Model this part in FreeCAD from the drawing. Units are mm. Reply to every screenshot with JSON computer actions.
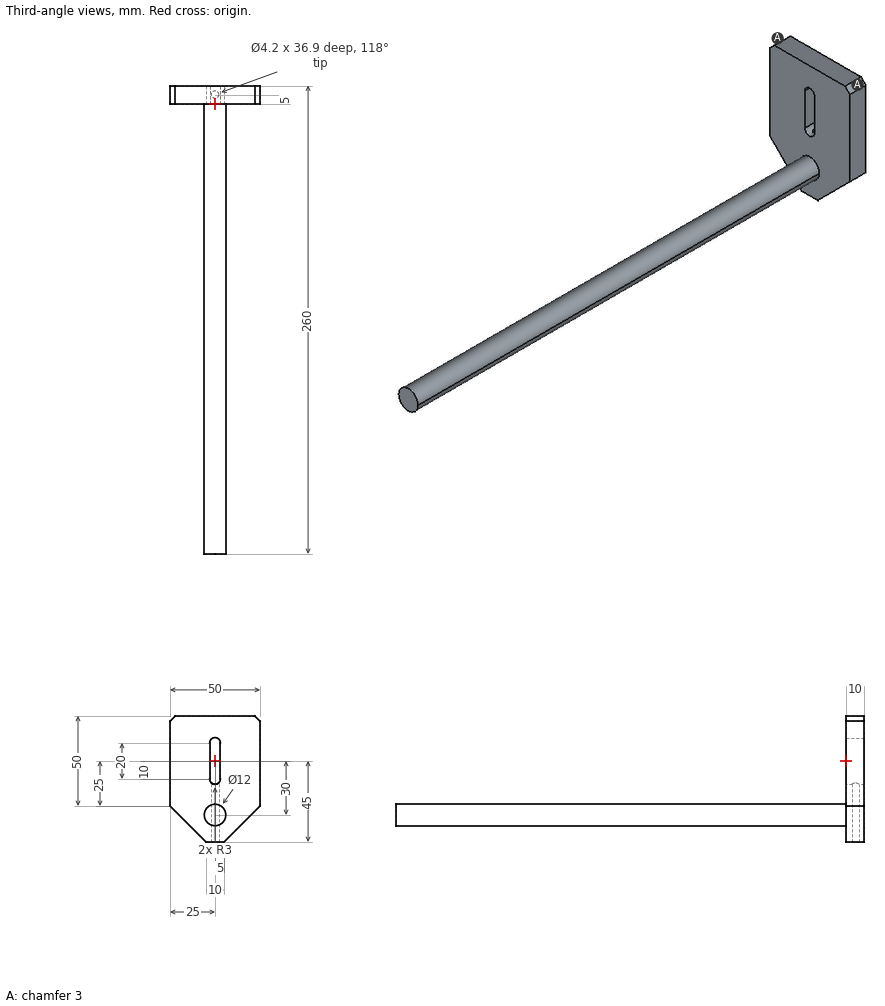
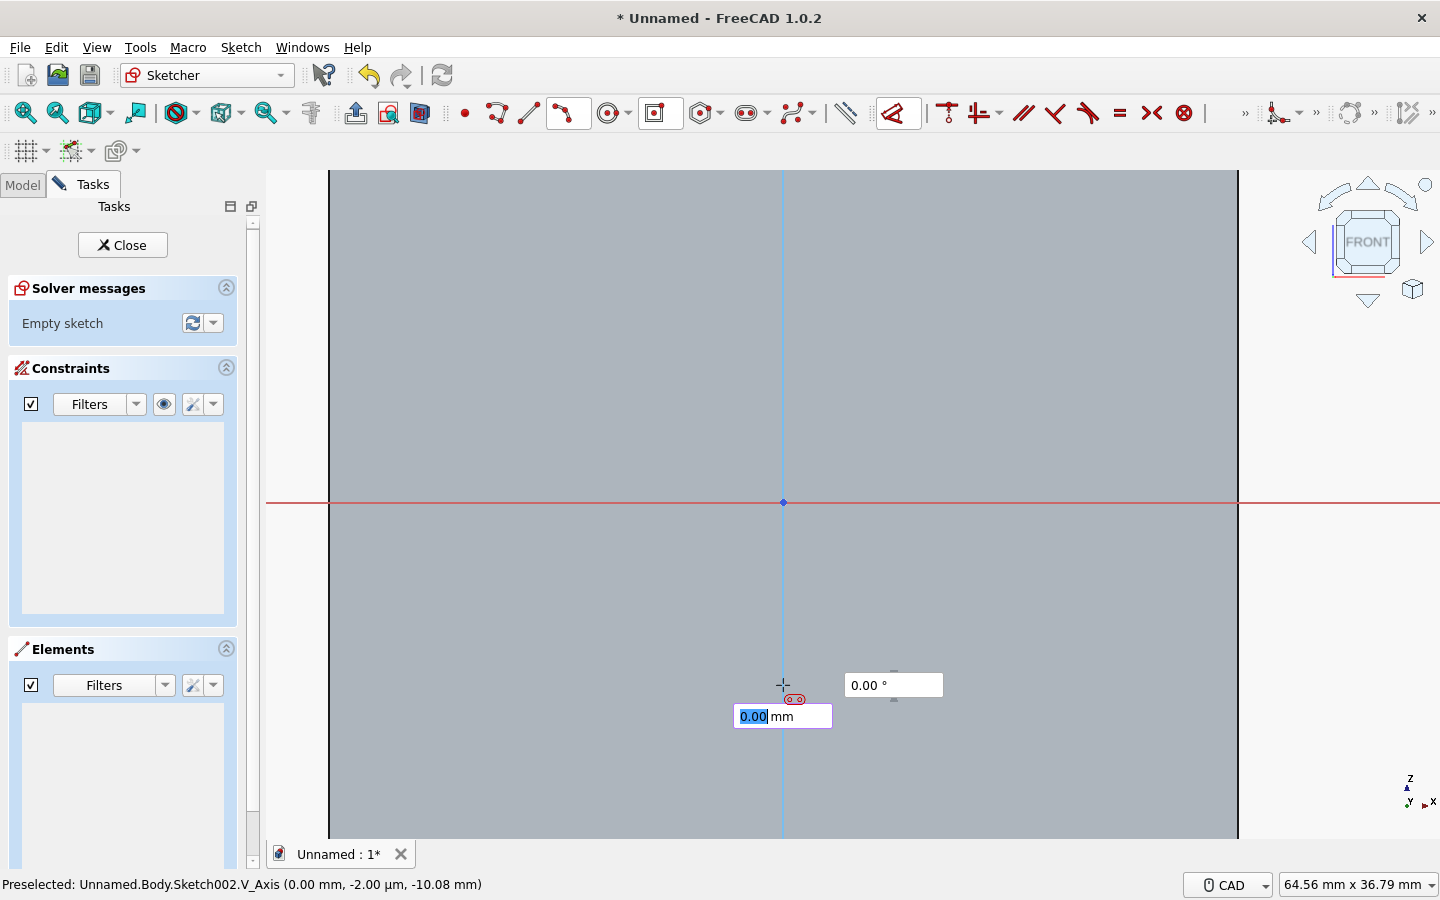
{"action": "left_click", "coordinate": [792, 321]}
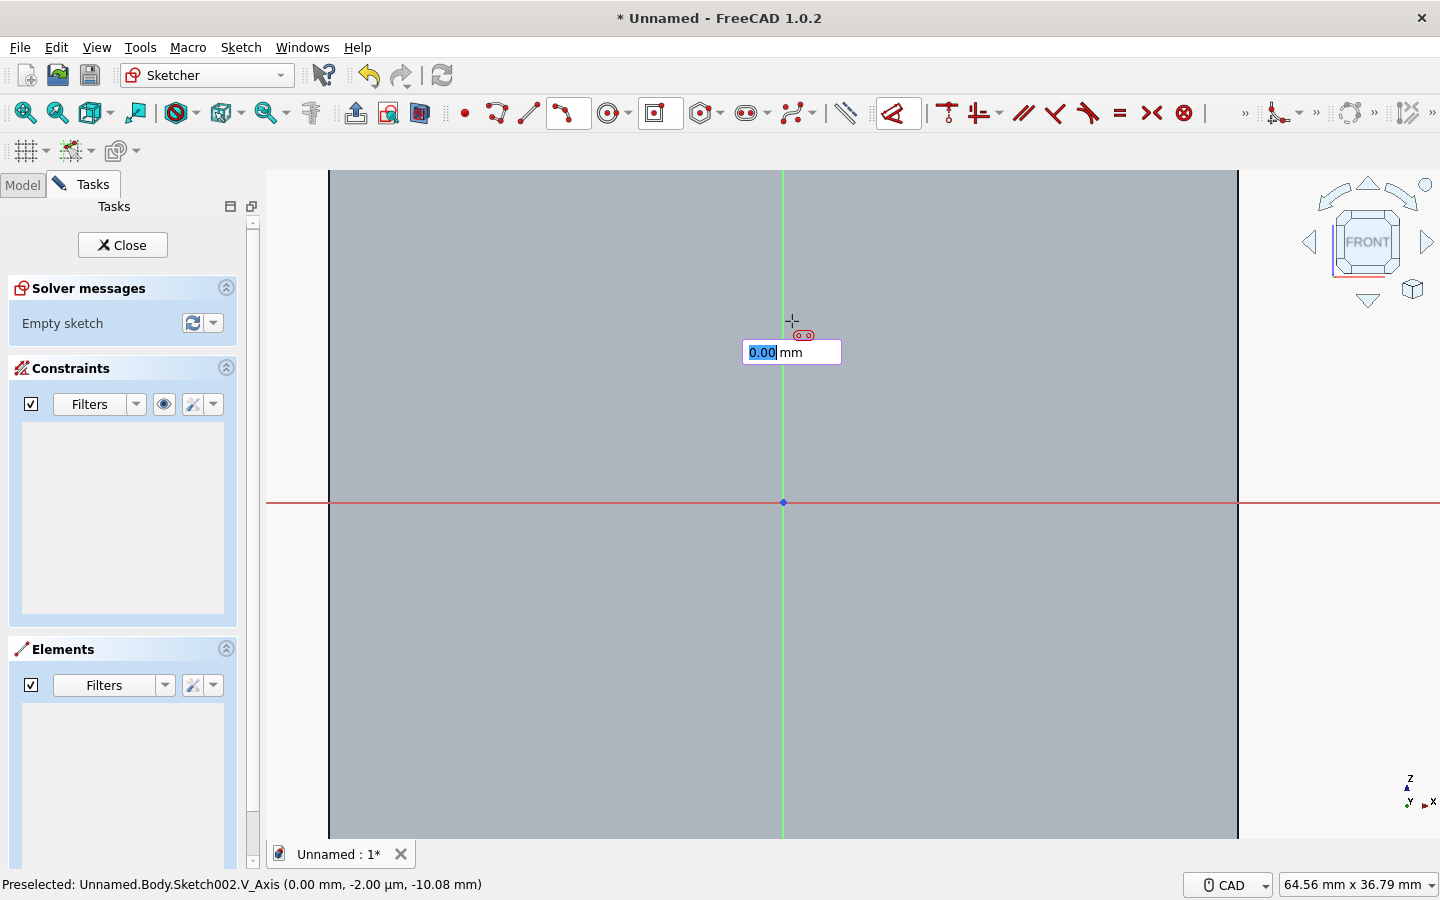
{"action": "left_click", "coordinate": [729, 448]}
{"action": "key", "text": "Escape"}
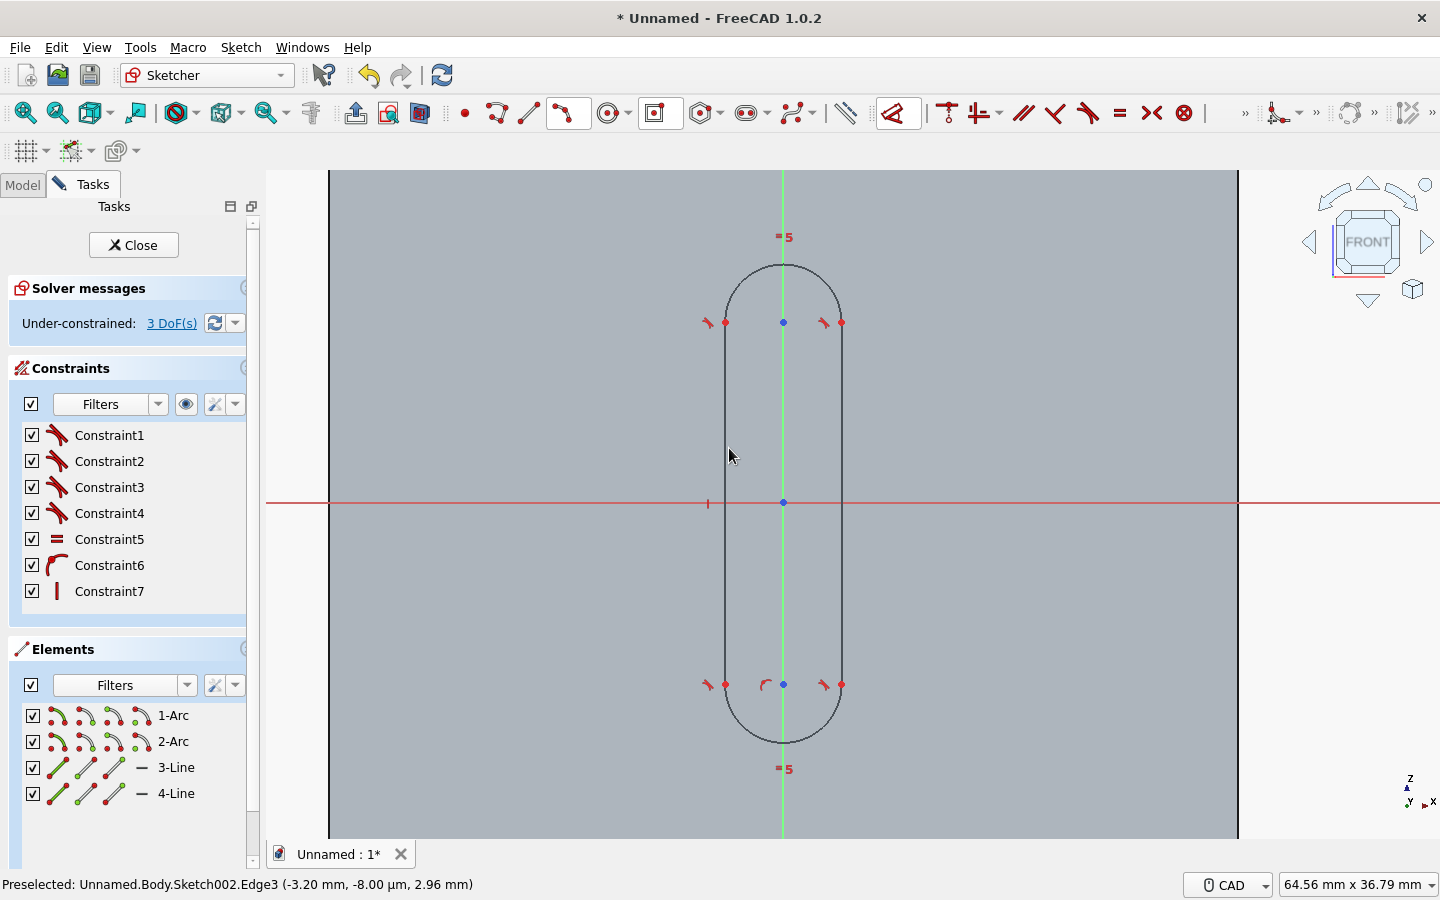
{"action": "left_click", "coordinate": [749, 732]}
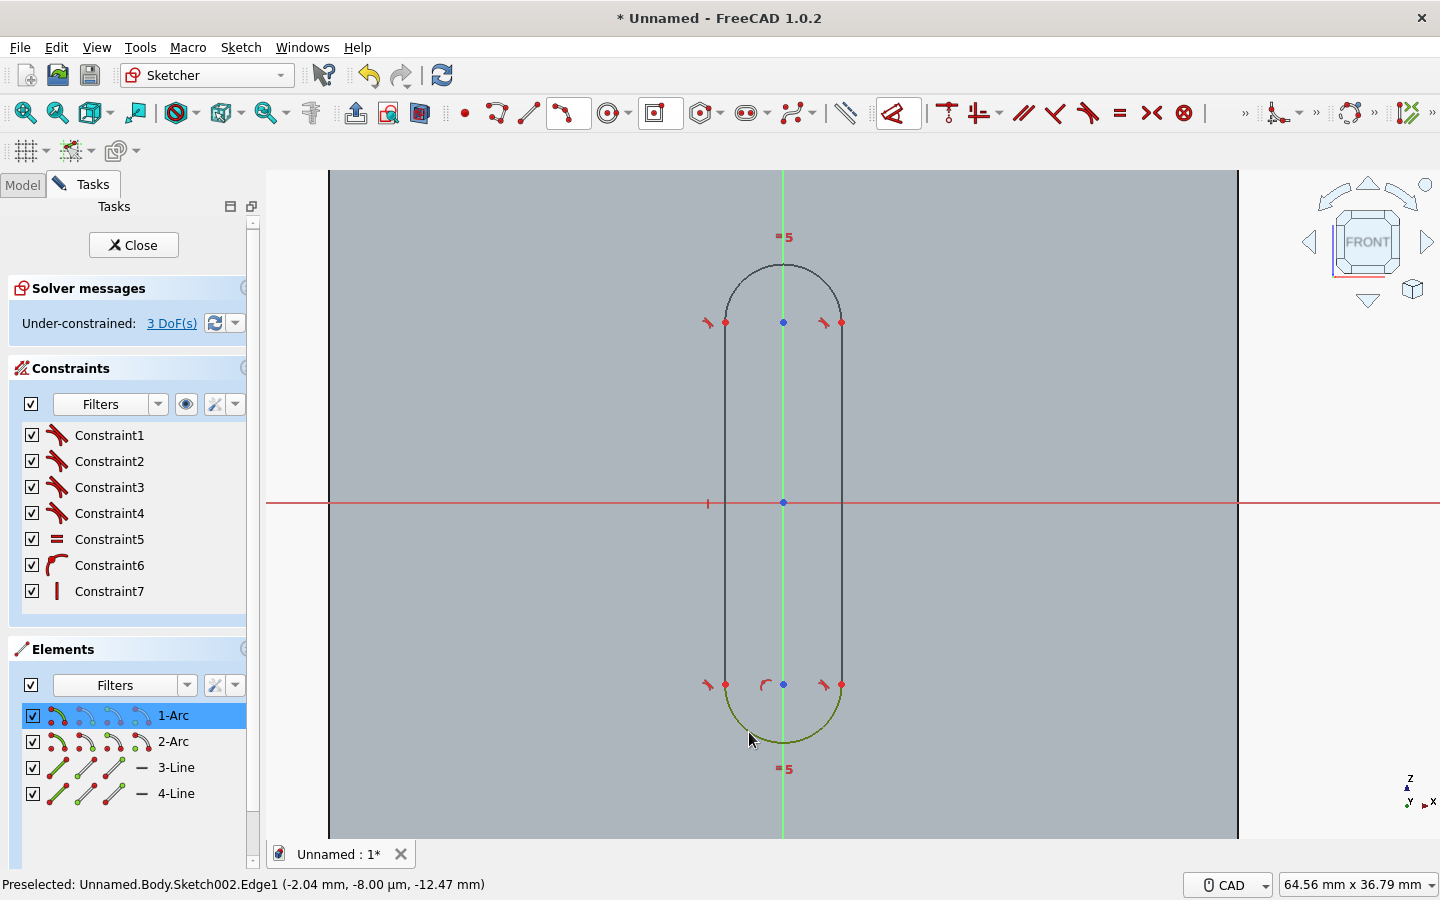
{"action": "key", "text": "k r"}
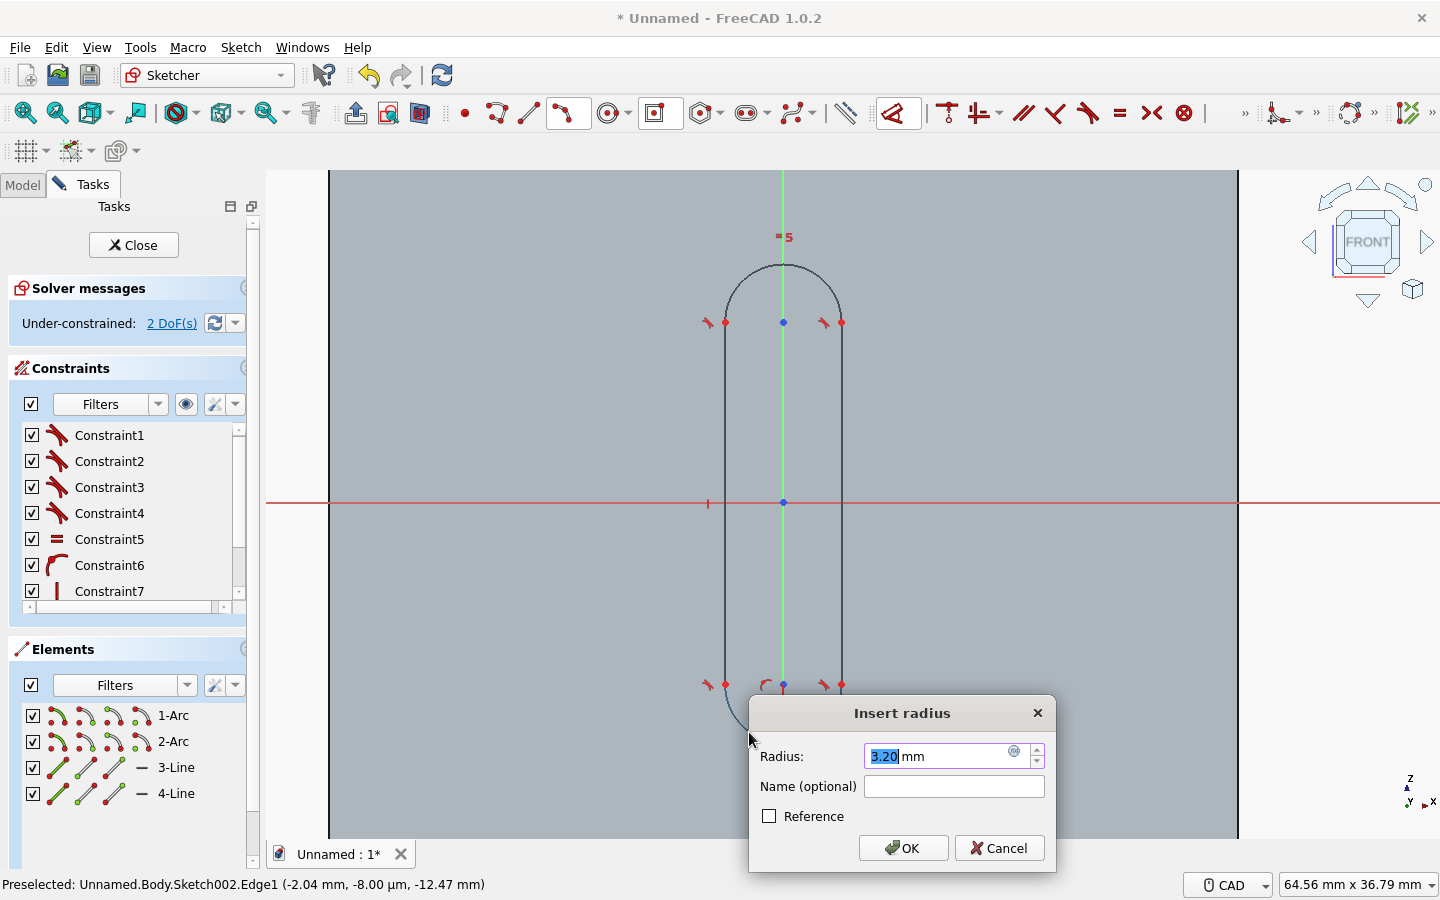
{"action": "type", "text": "3"}
{"action": "key", "text": "Return"}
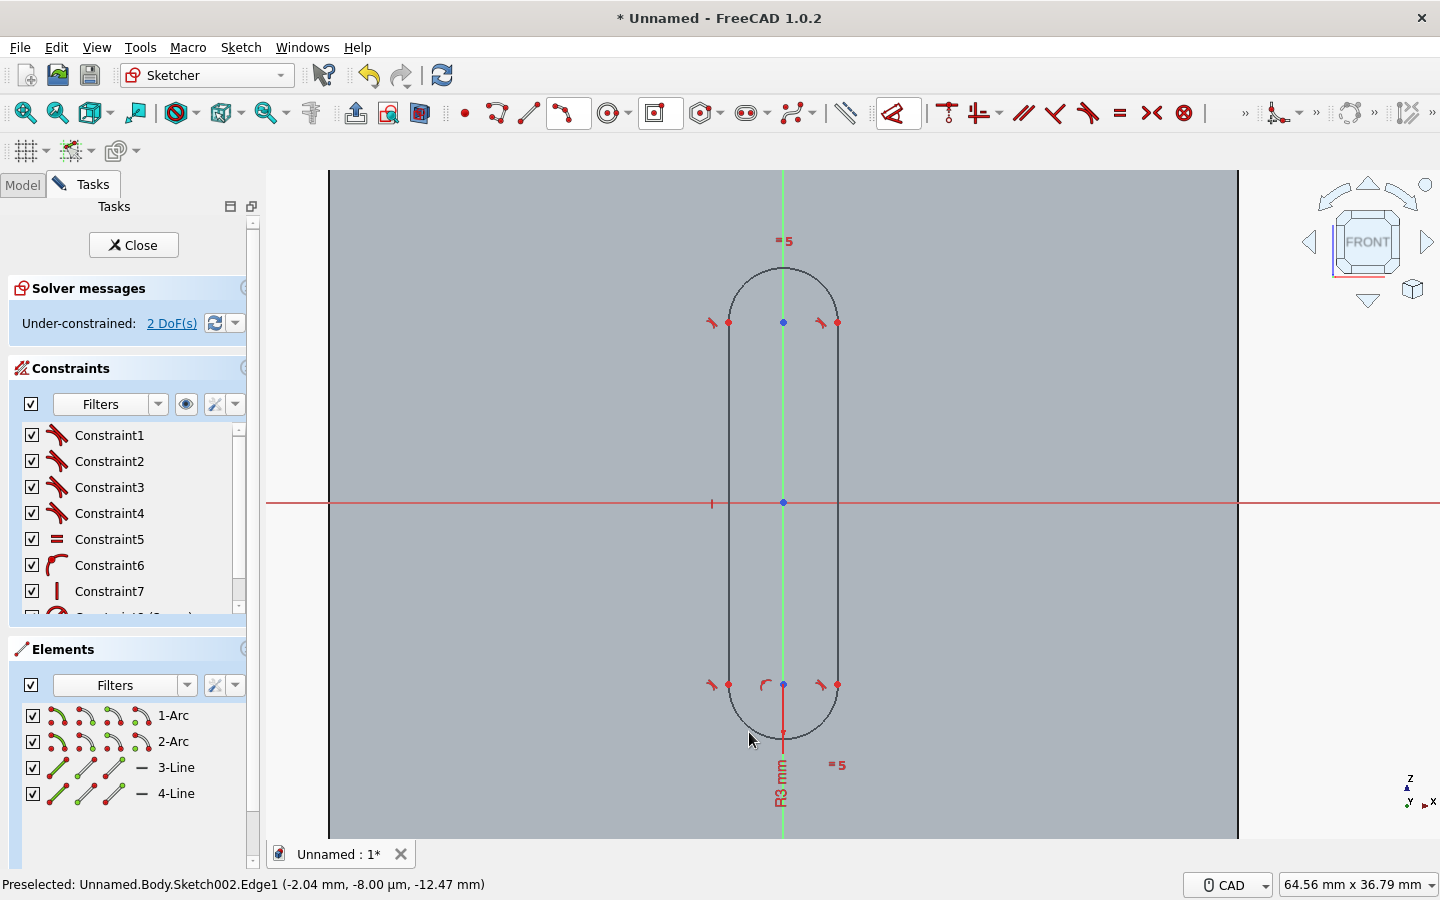
{"action": "left_click", "coordinate": [729, 576]}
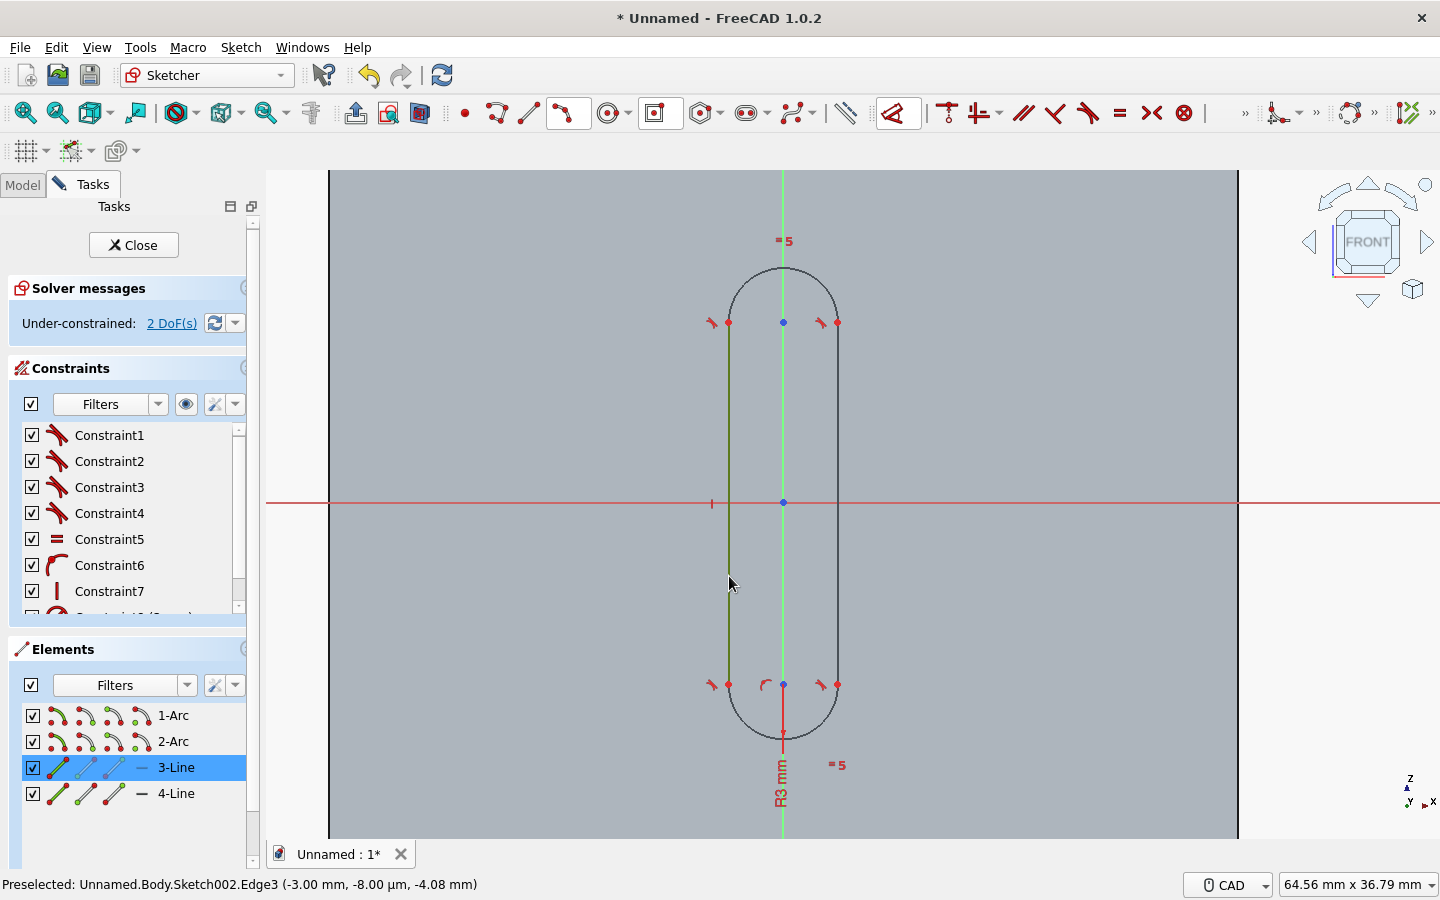
{"action": "key", "text": "i"}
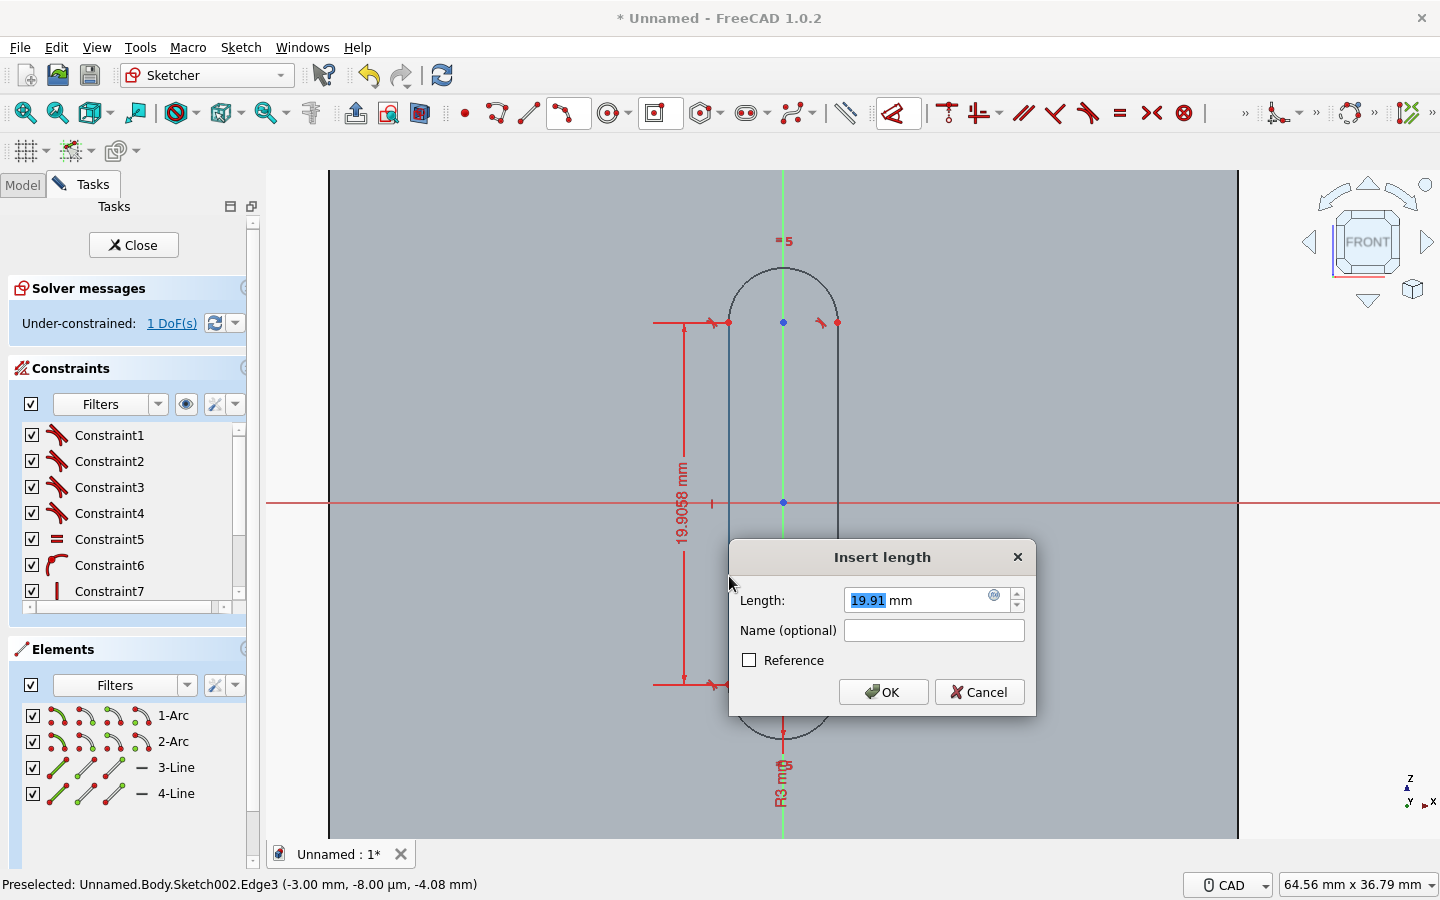
{"action": "type", "text": "20"}
{"action": "key", "text": "Return"}